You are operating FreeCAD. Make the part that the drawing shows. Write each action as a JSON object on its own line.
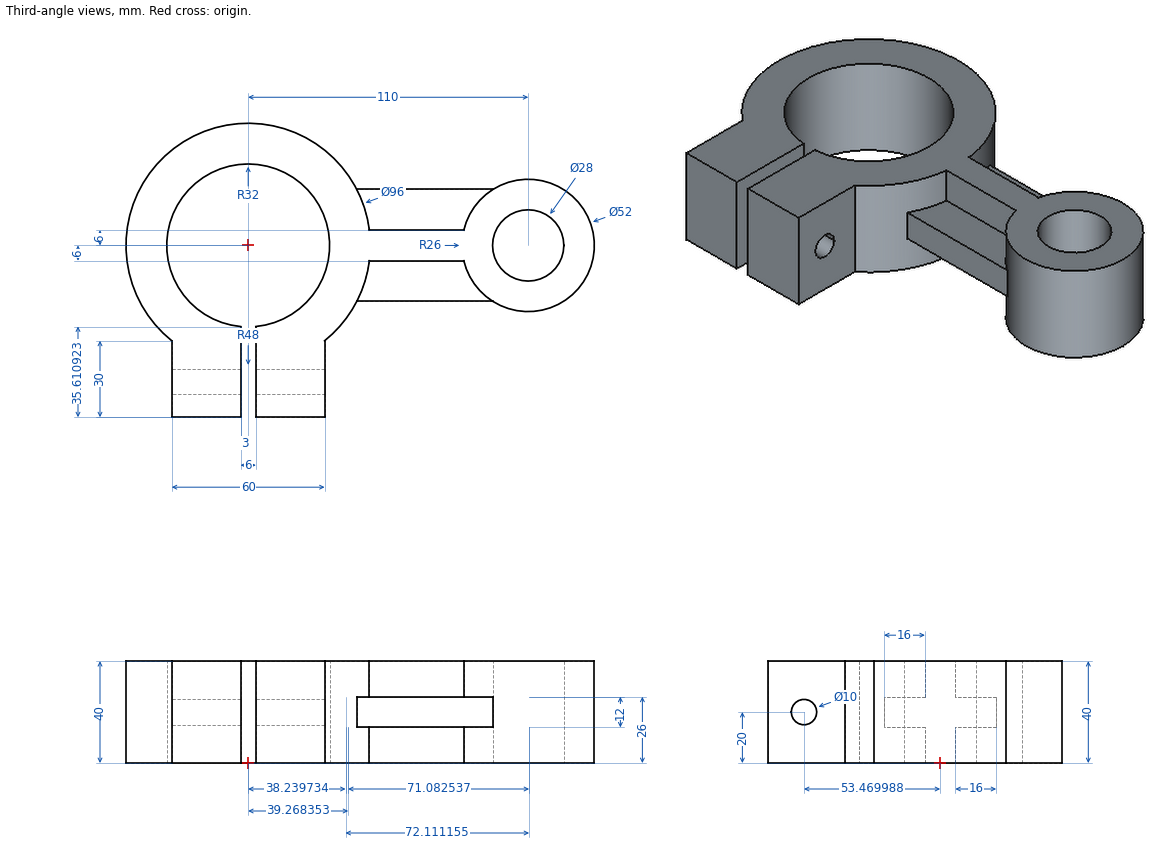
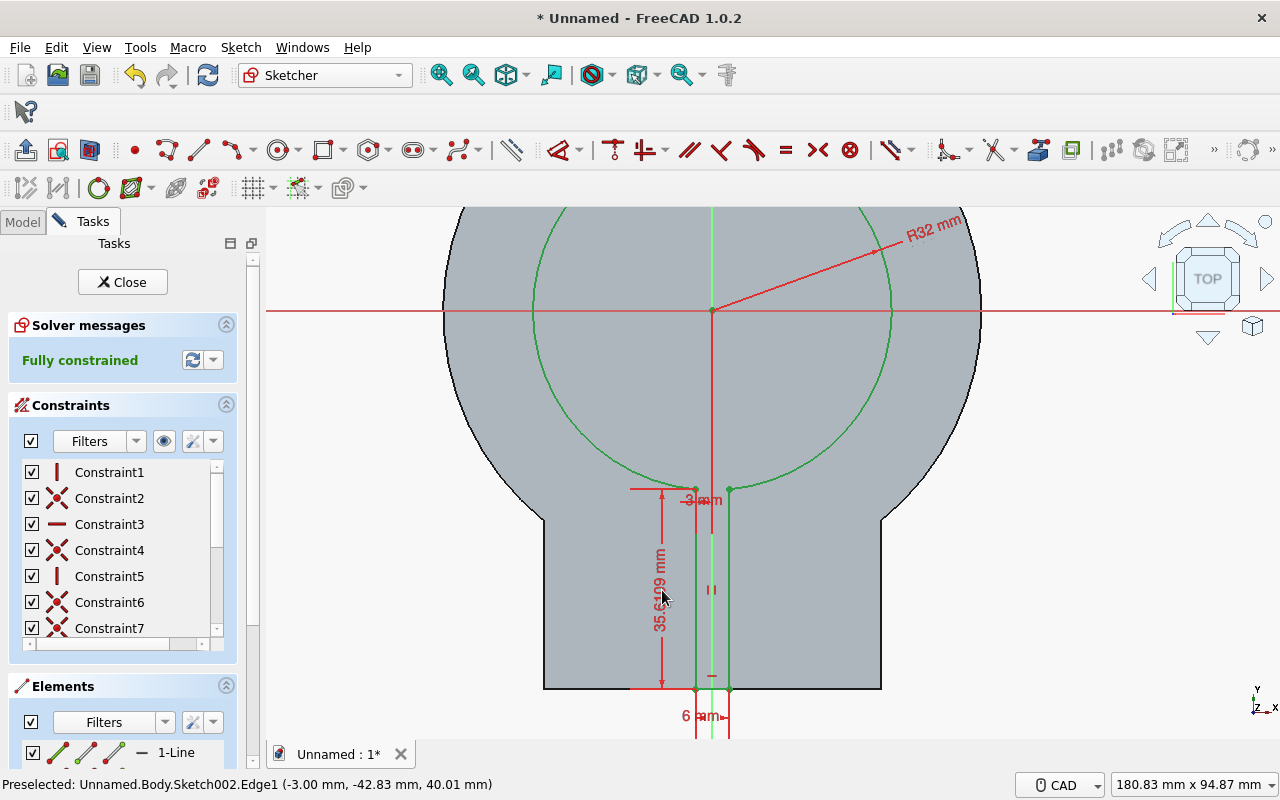
{"action": "left_click", "coordinate": [123, 282]}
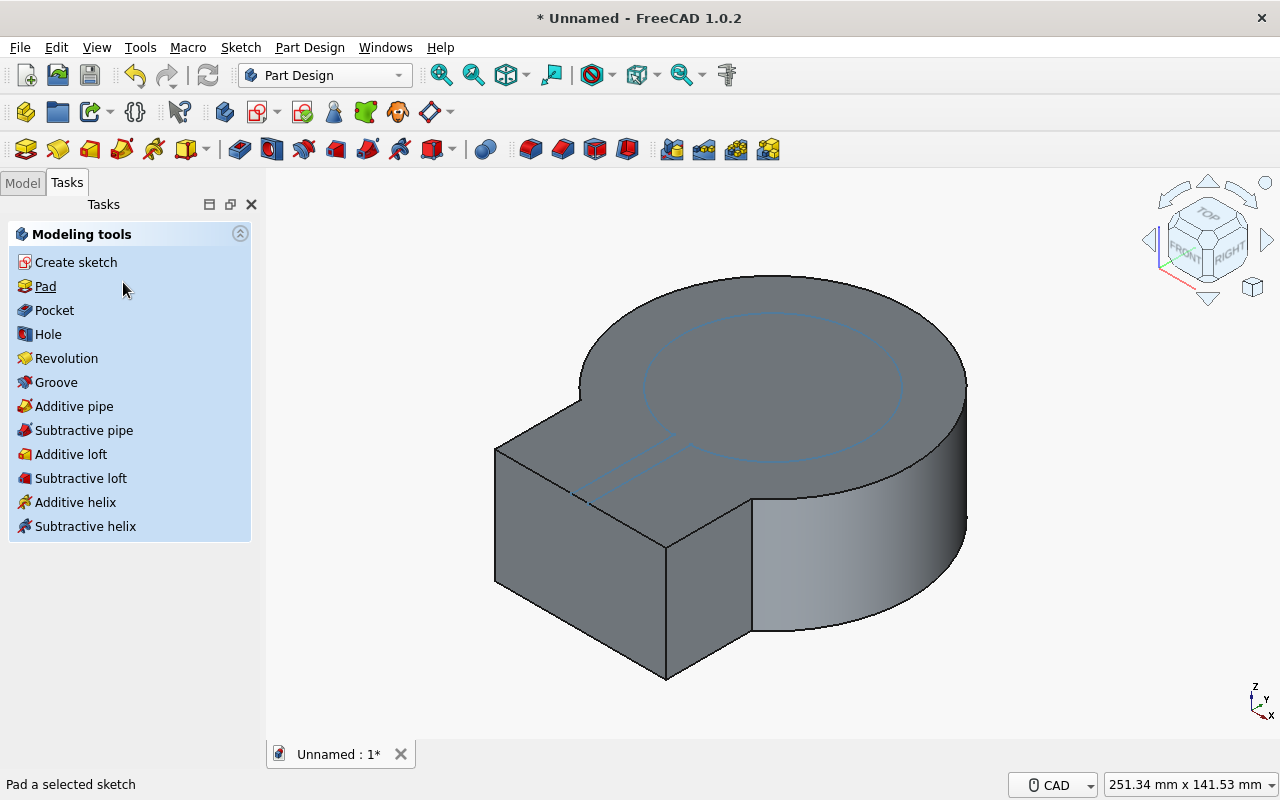
{"action": "left_click", "coordinate": [240, 150]}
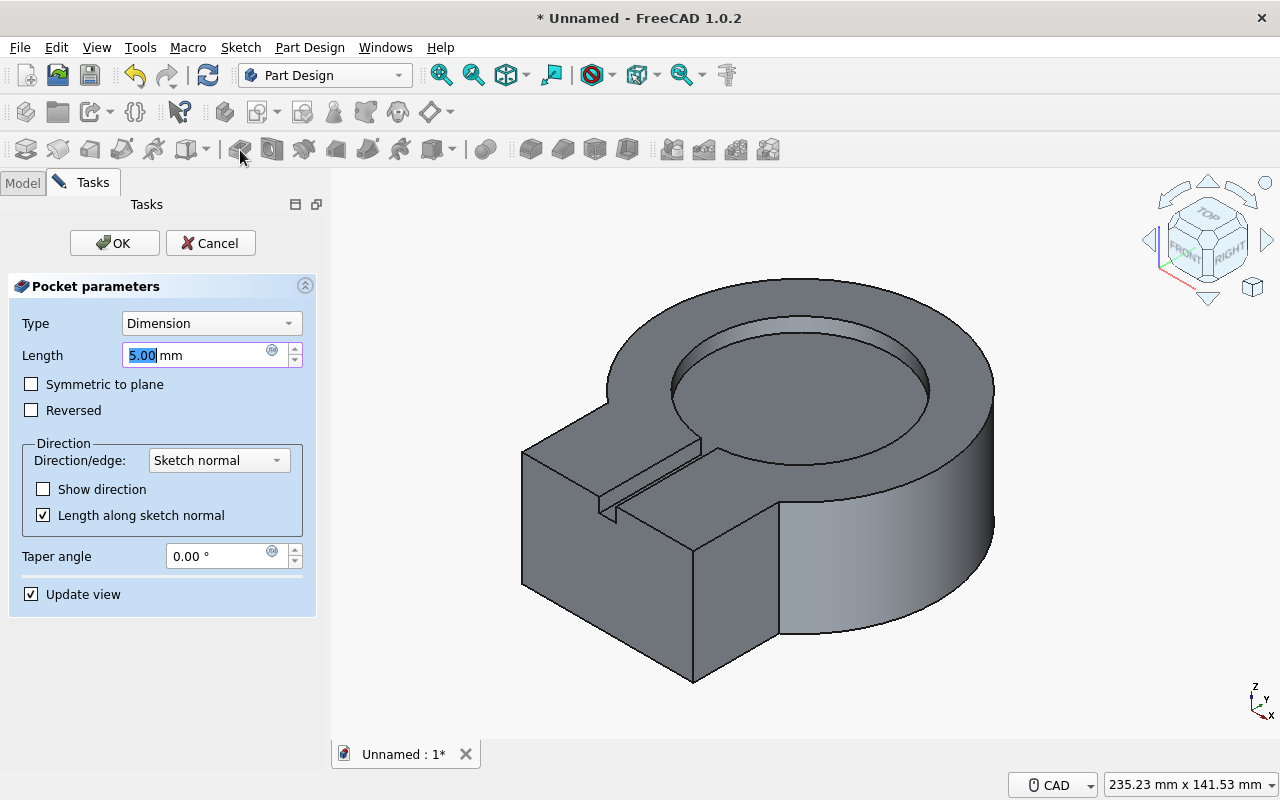
{"action": "type", "text": "40"}
{"action": "key", "text": "Tab"}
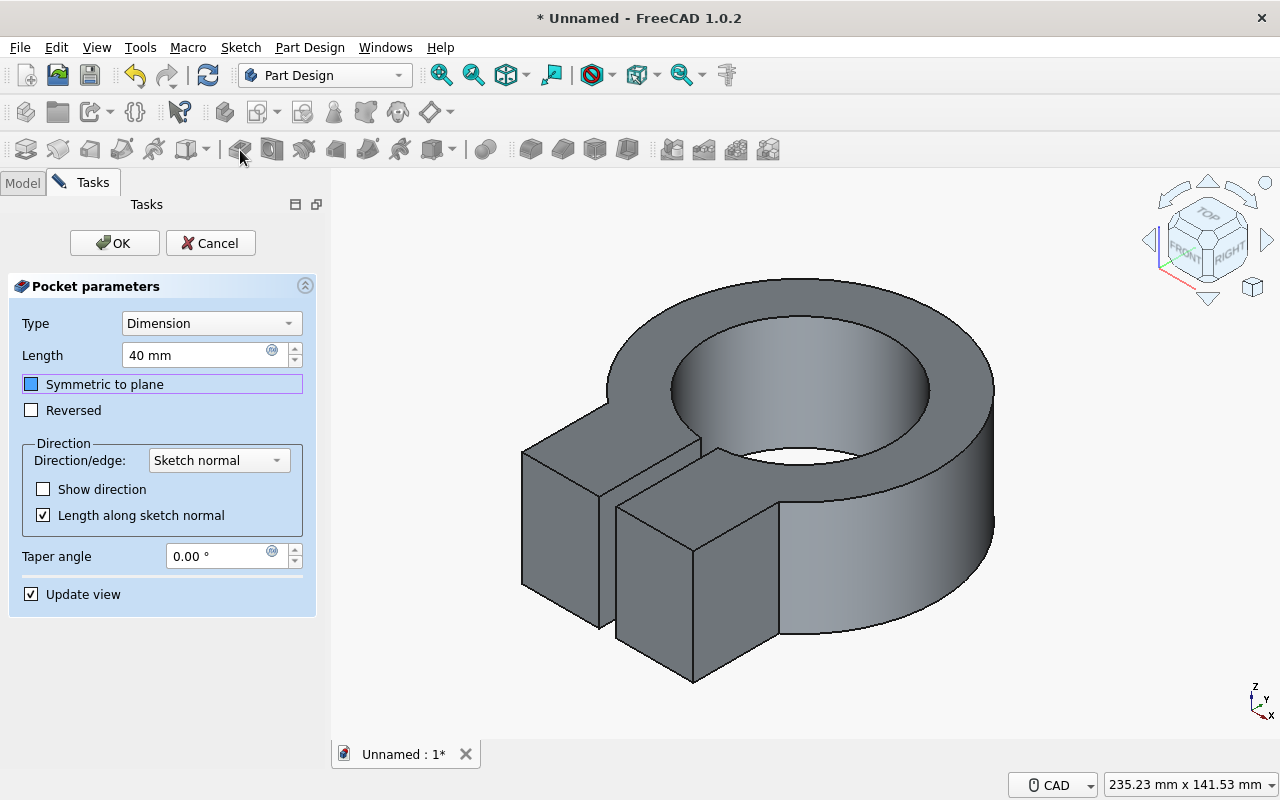
{"action": "left_click", "coordinate": [115, 243]}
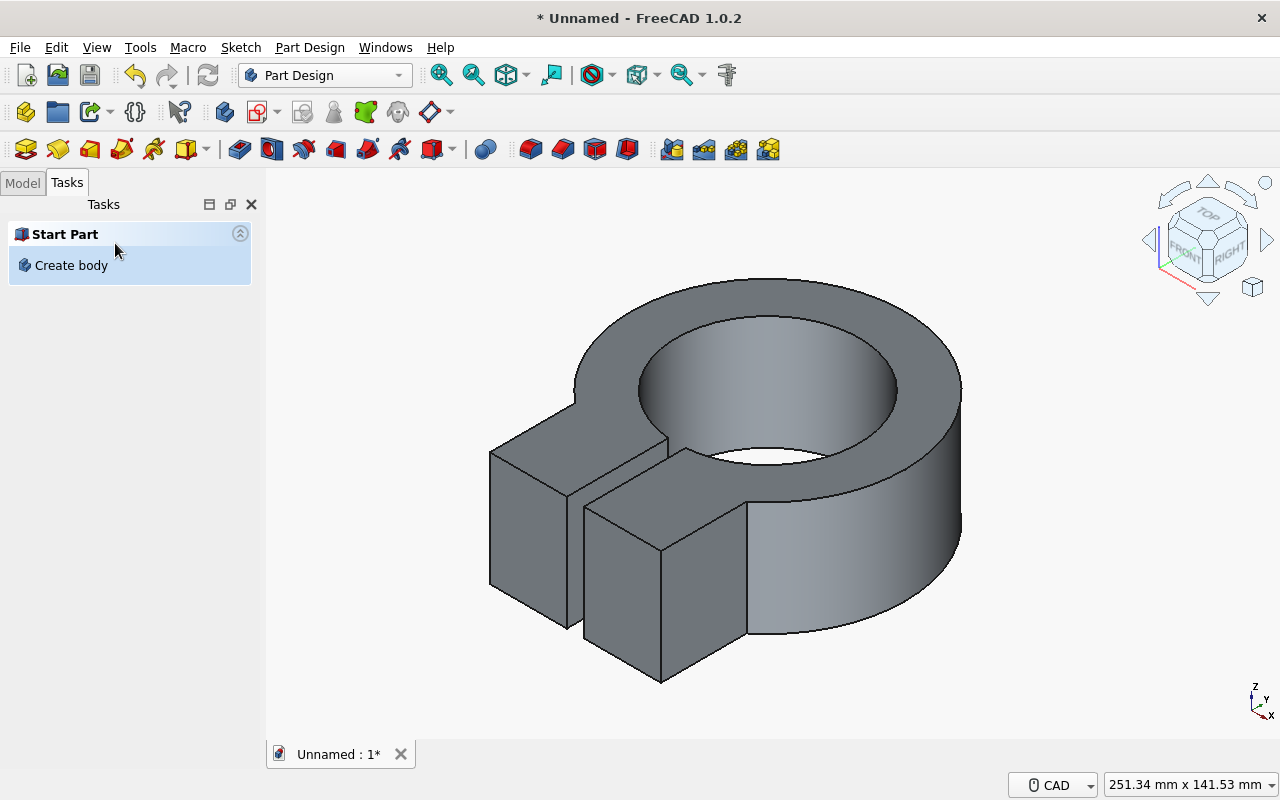
{"action": "left_click", "coordinate": [226, 112]}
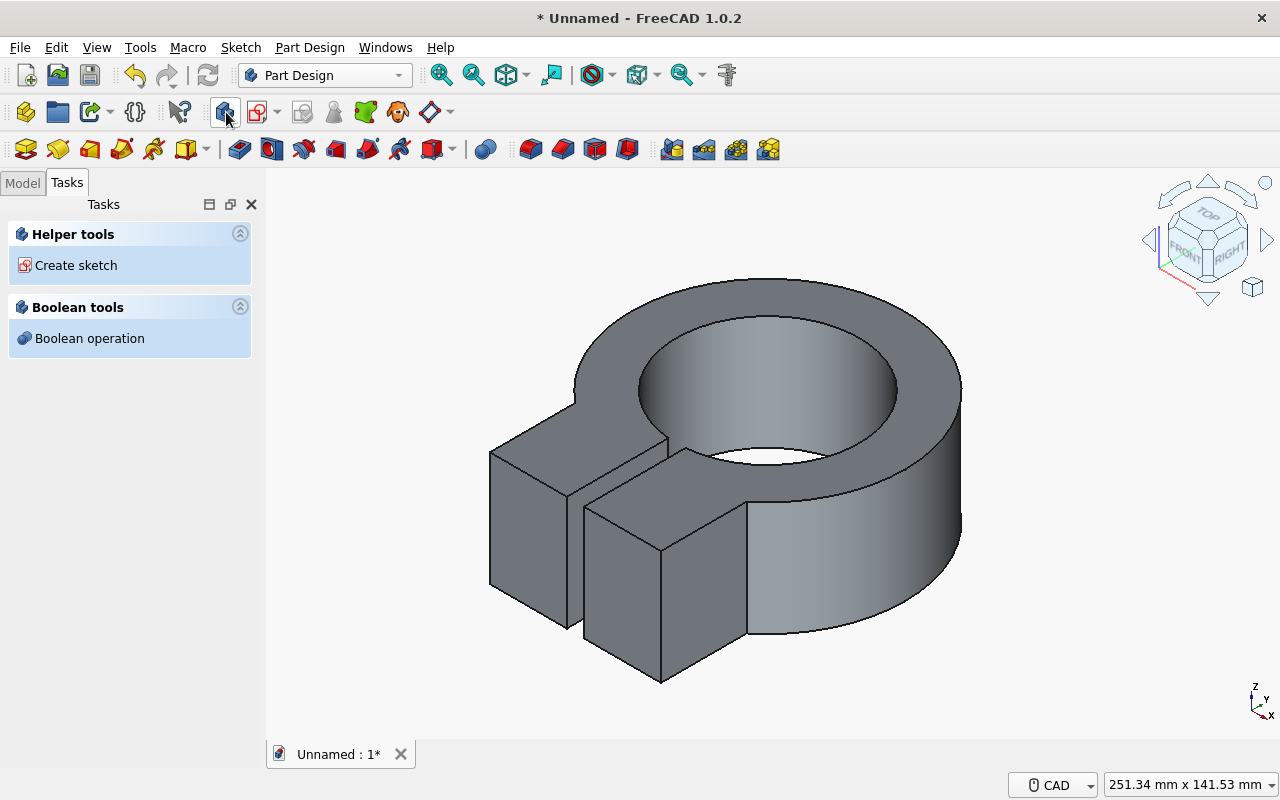
{"action": "left_click", "coordinate": [23, 182]}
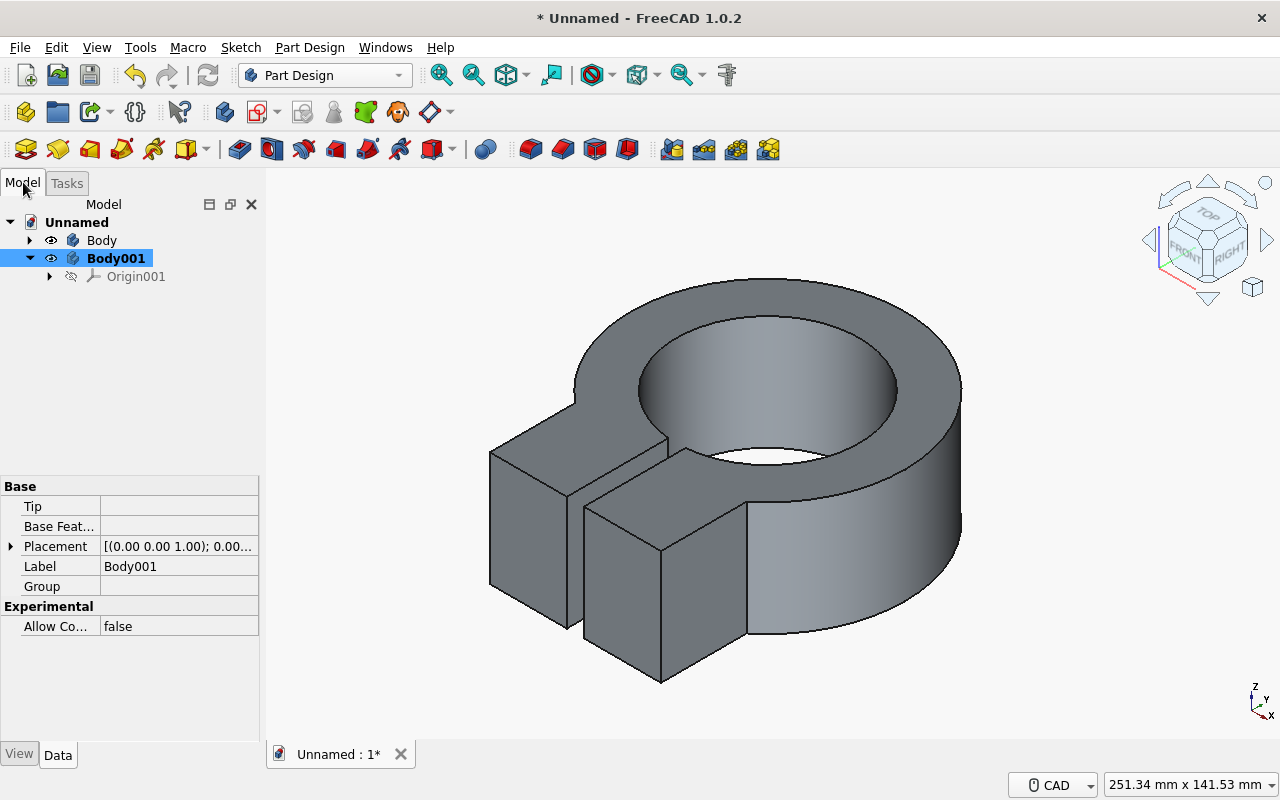
{"action": "left_click", "coordinate": [50, 276]}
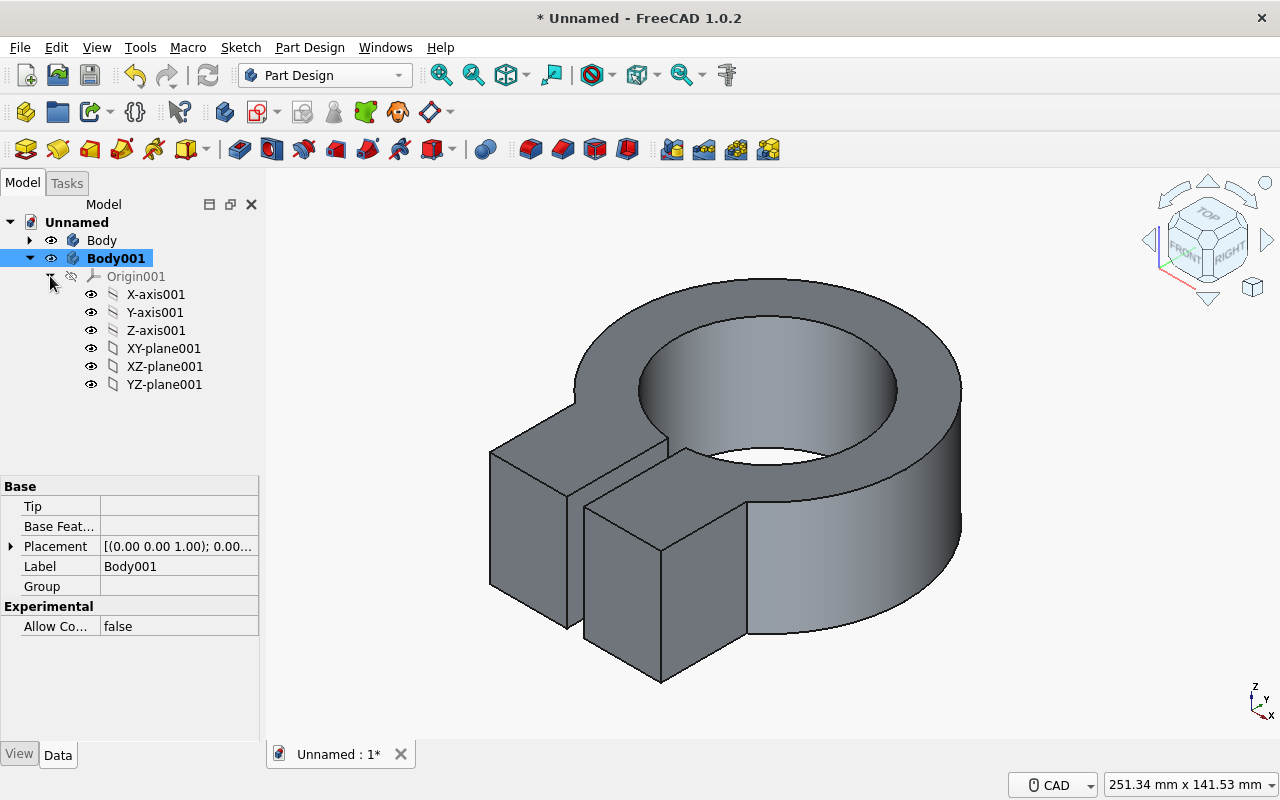
{"action": "left_click", "coordinate": [136, 348]}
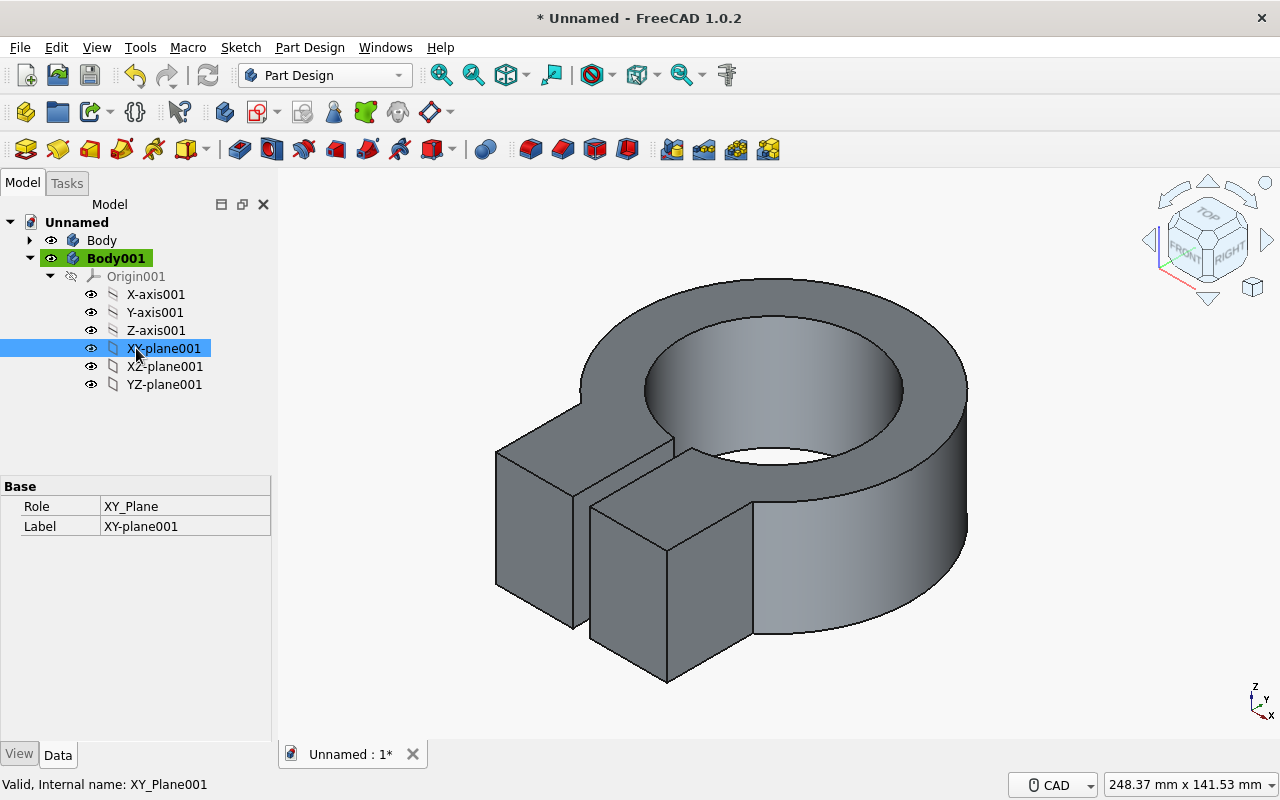
{"action": "left_click", "coordinate": [430, 112]}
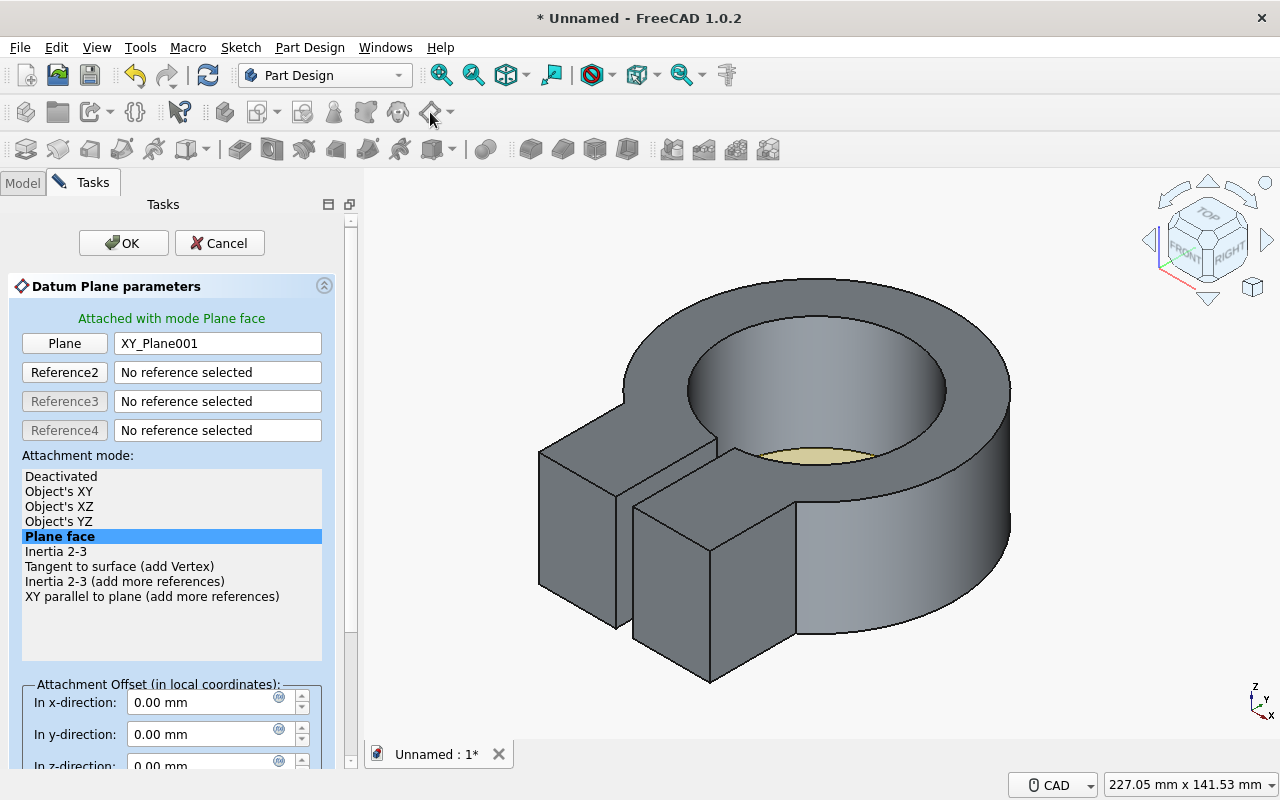
{"action": "scroll", "coordinate": [351, 491], "scroll_direction": "down", "scroll_amount": 2}